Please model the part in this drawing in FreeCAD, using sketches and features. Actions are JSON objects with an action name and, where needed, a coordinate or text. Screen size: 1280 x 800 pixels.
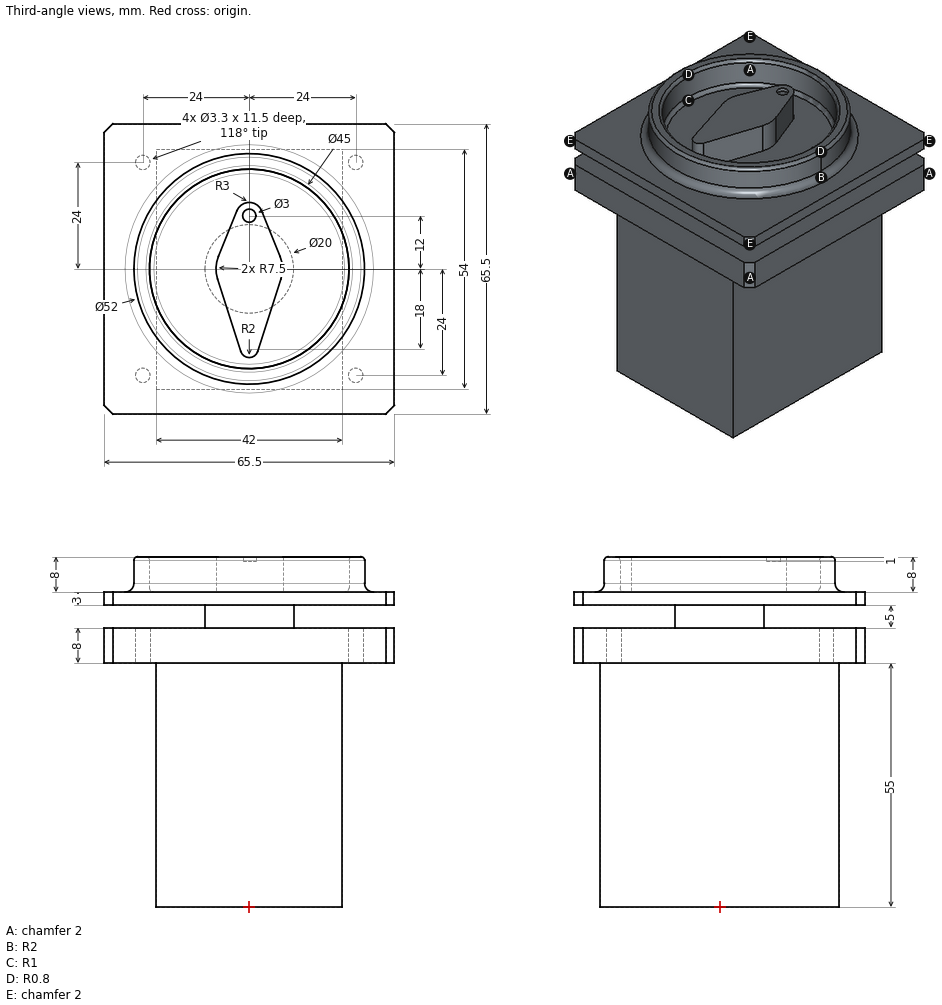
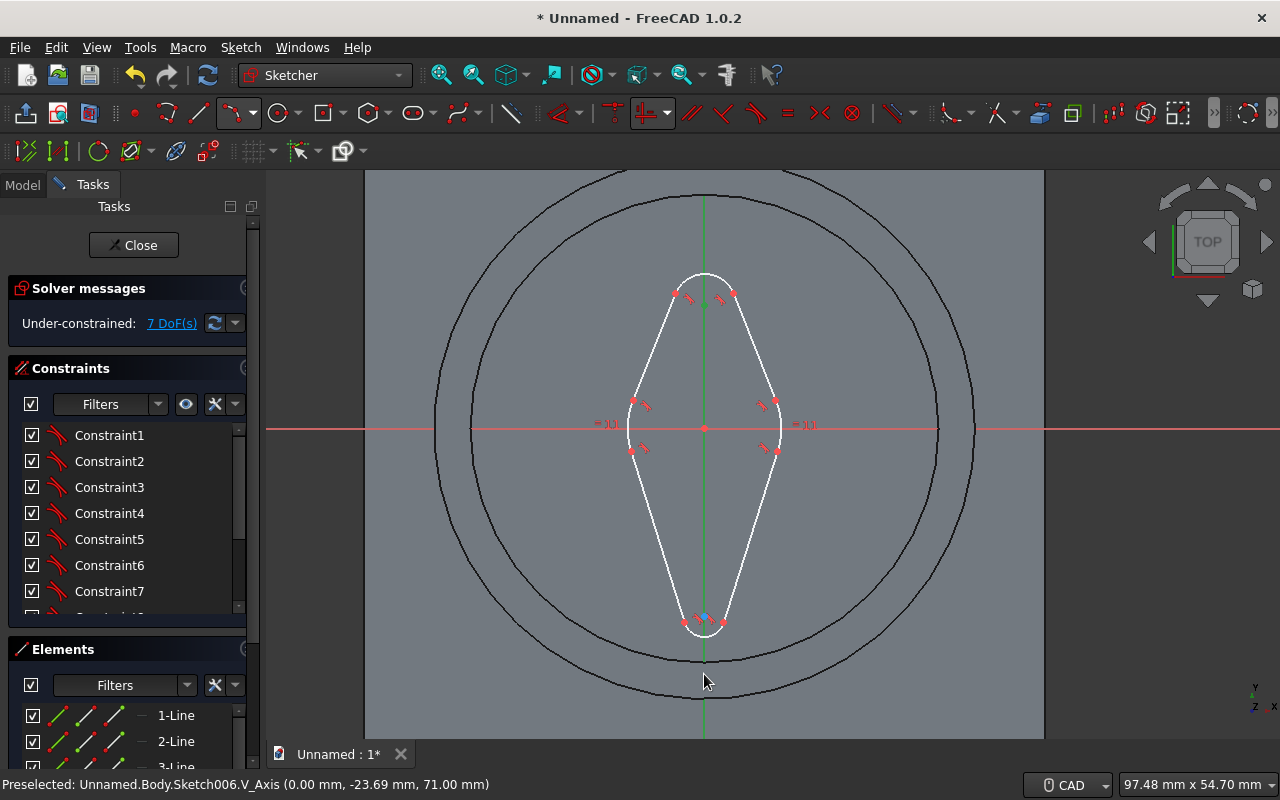
{"action": "left_click", "coordinate": [614, 114]}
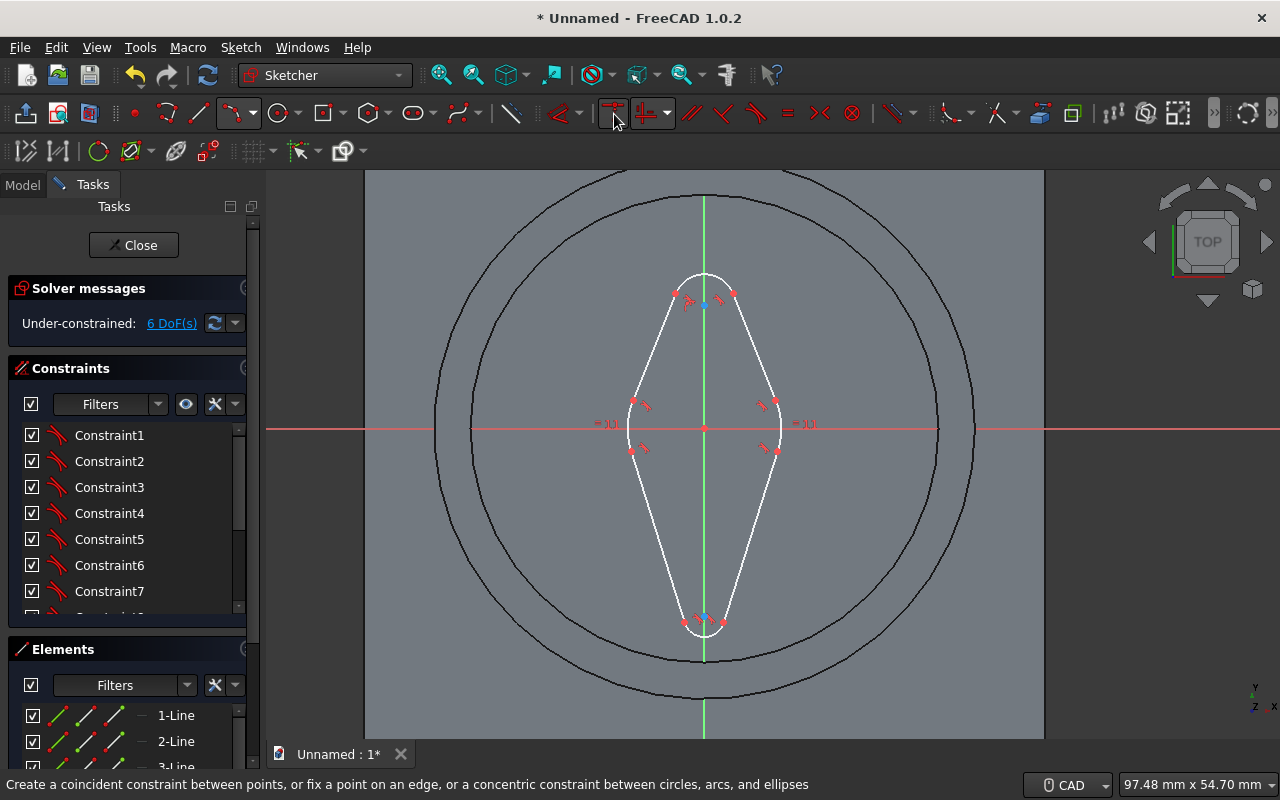
{"action": "left_click", "coordinate": [704, 617]}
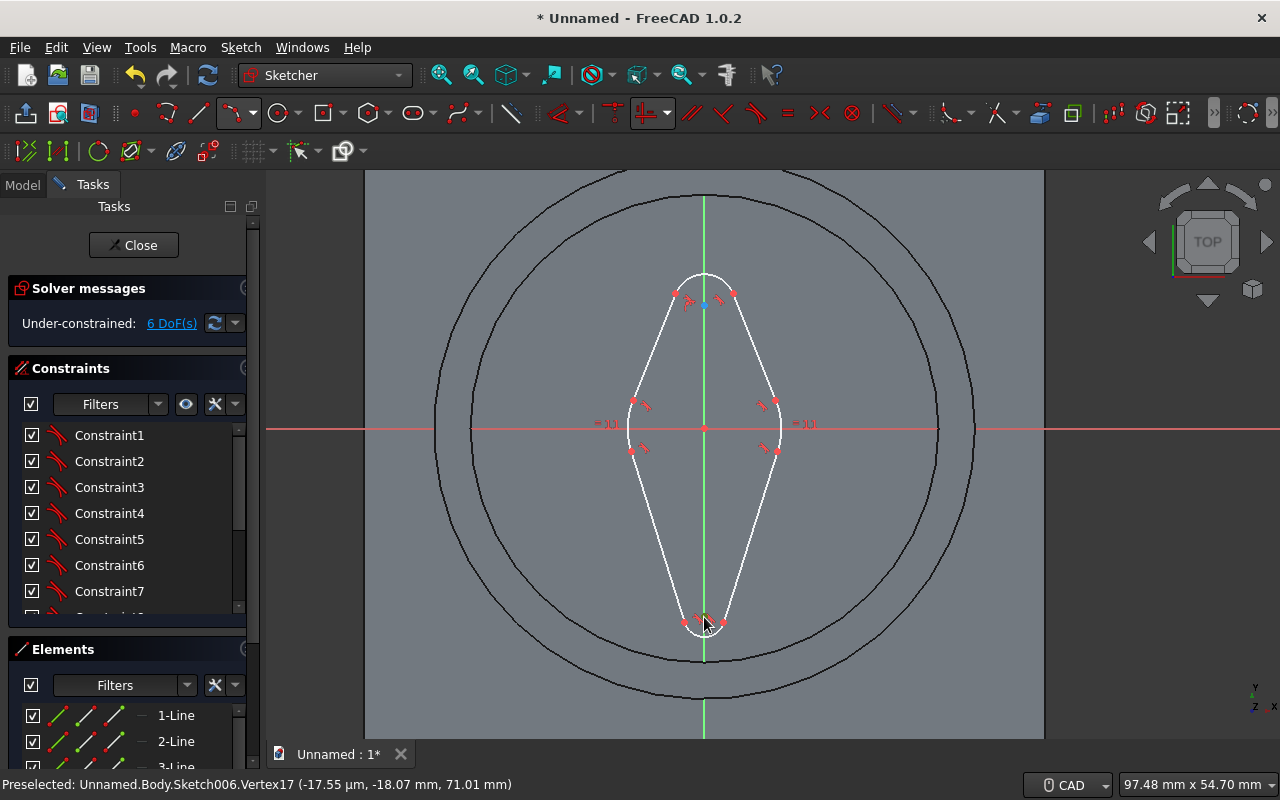
{"action": "left_click", "coordinate": [704, 674]}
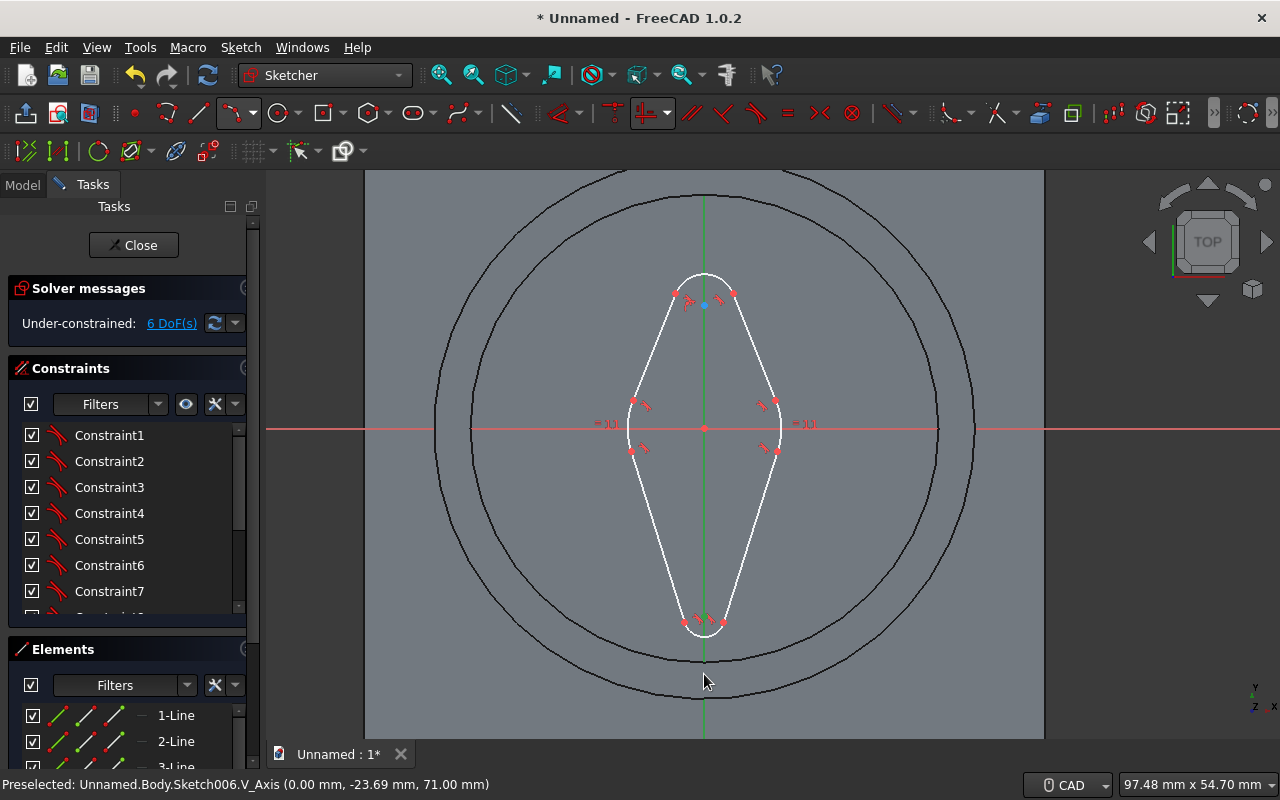
{"action": "left_click", "coordinate": [614, 114]}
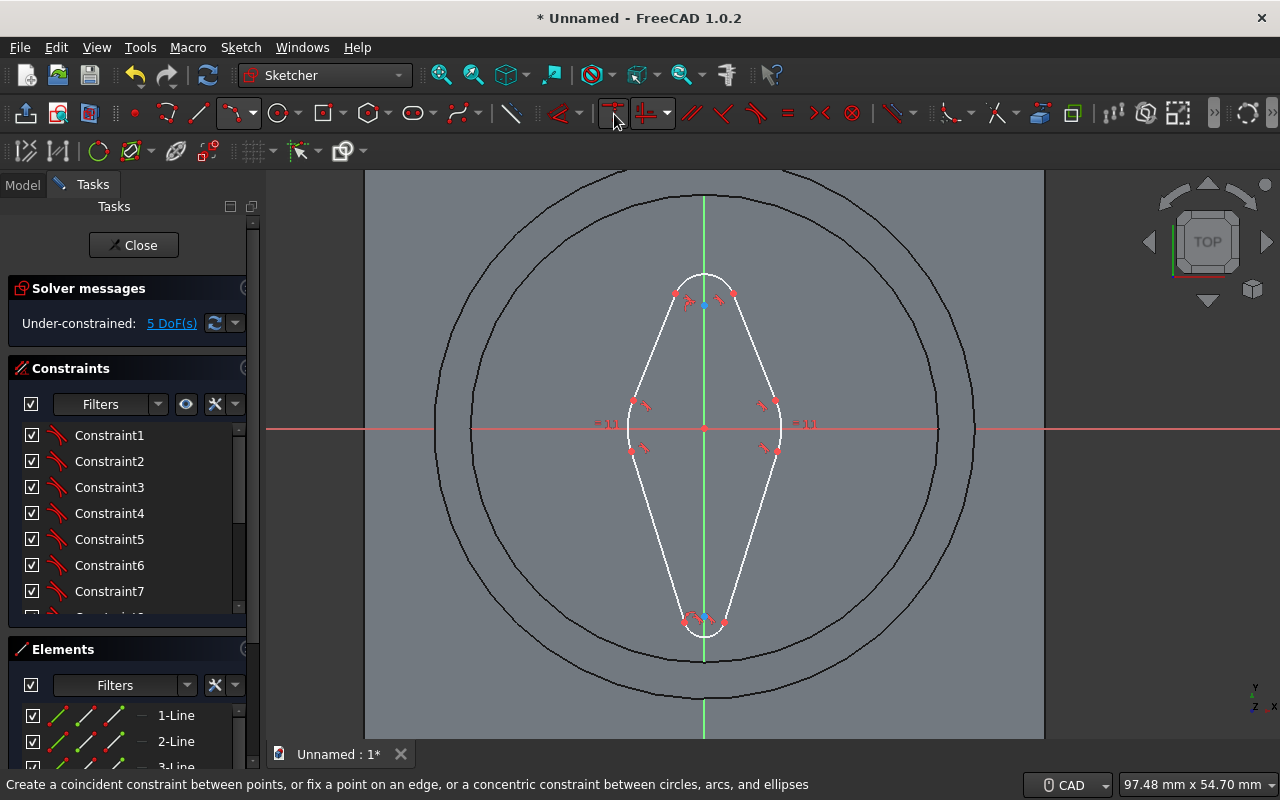
{"action": "left_click", "coordinate": [558, 114]}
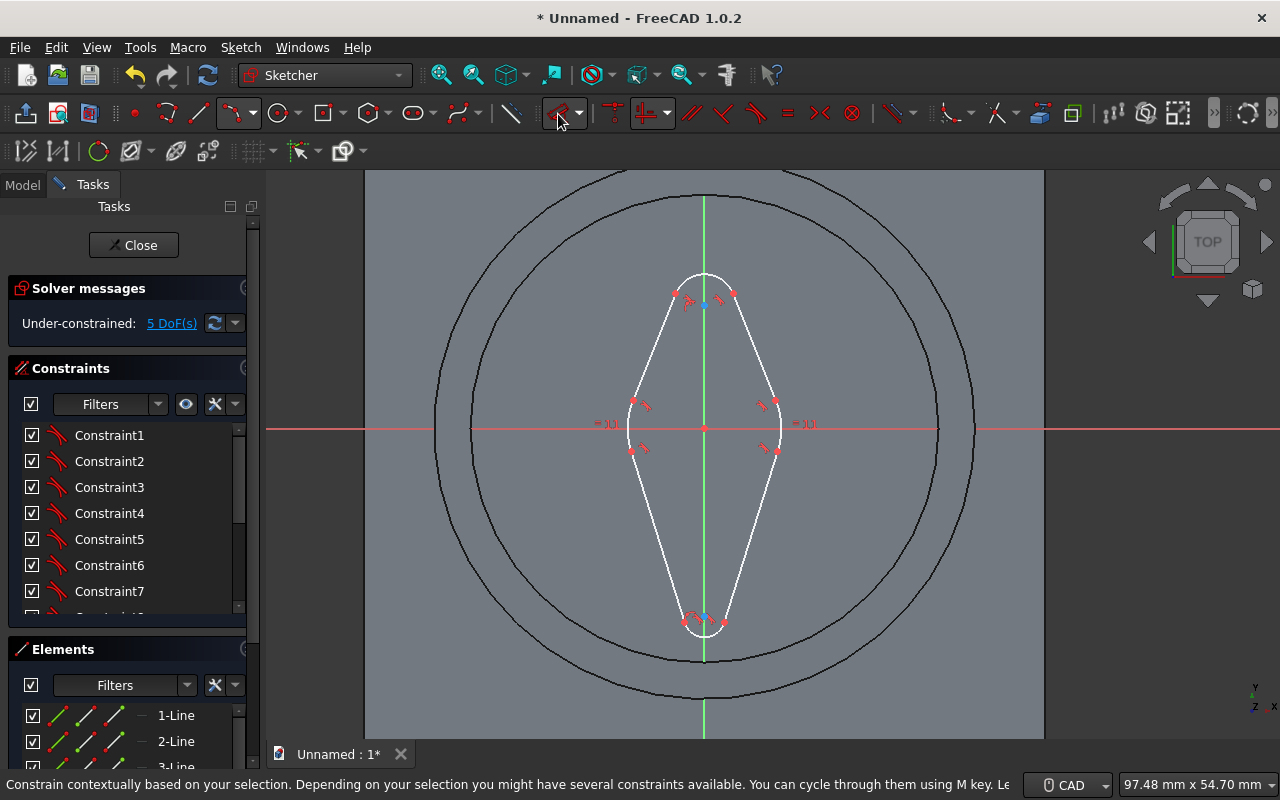
{"action": "scroll", "coordinate": [719, 278], "scroll_direction": "up", "scroll_amount": 2}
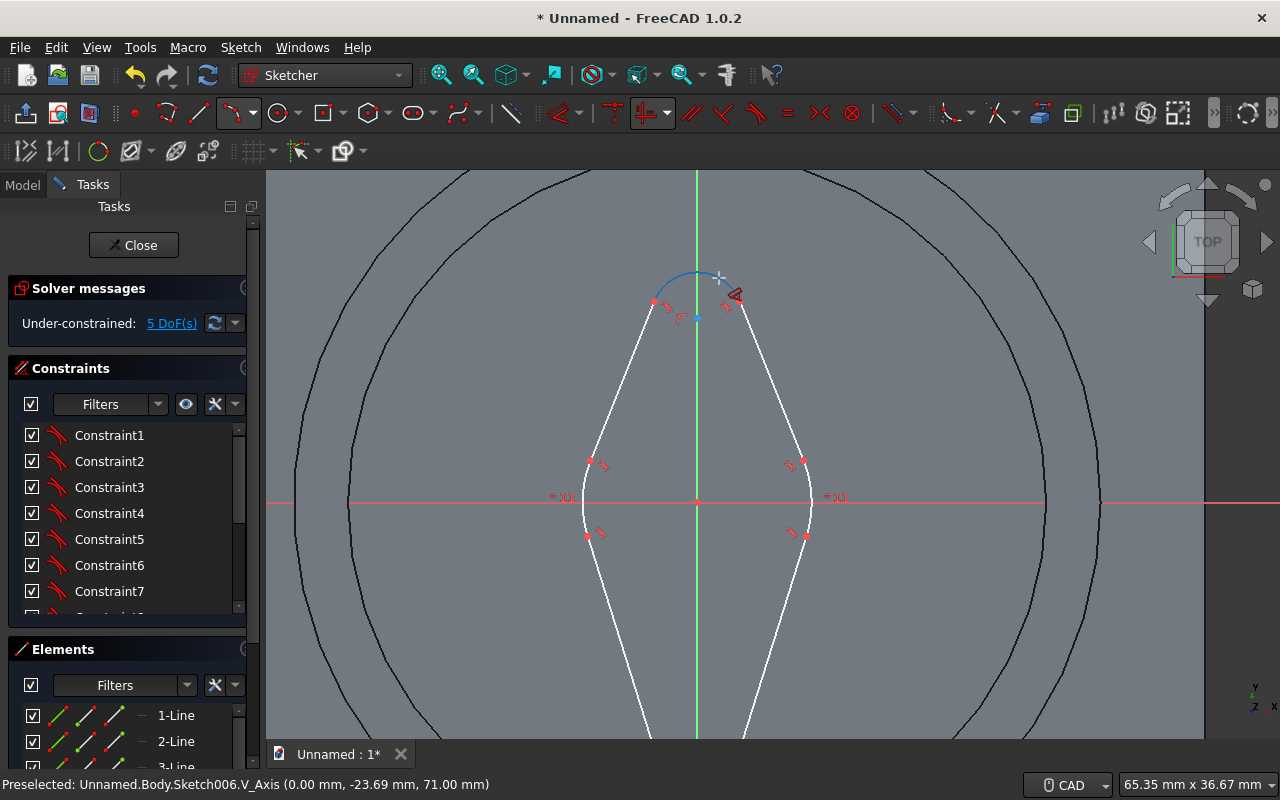
{"action": "left_click", "coordinate": [718, 278]}
{"action": "left_click", "coordinate": [733, 250]}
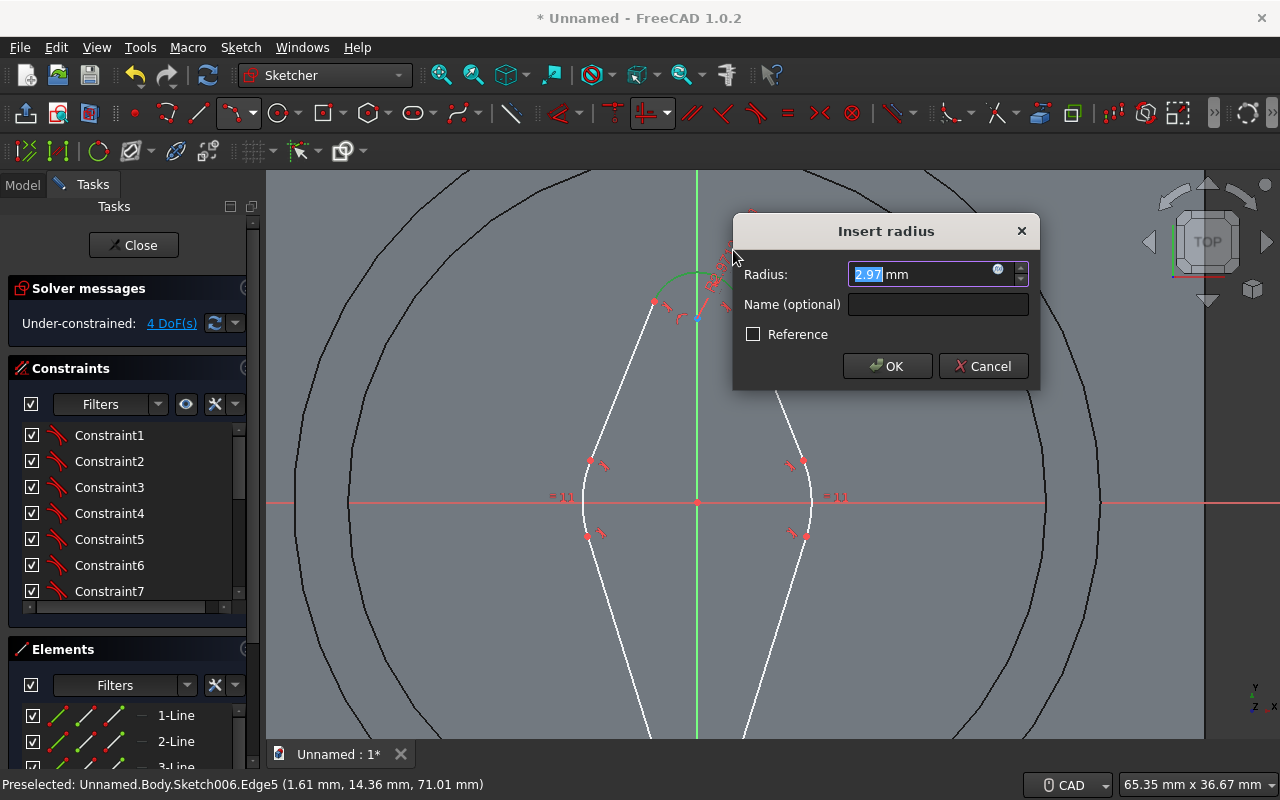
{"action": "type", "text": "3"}
{"action": "key", "text": "Return"}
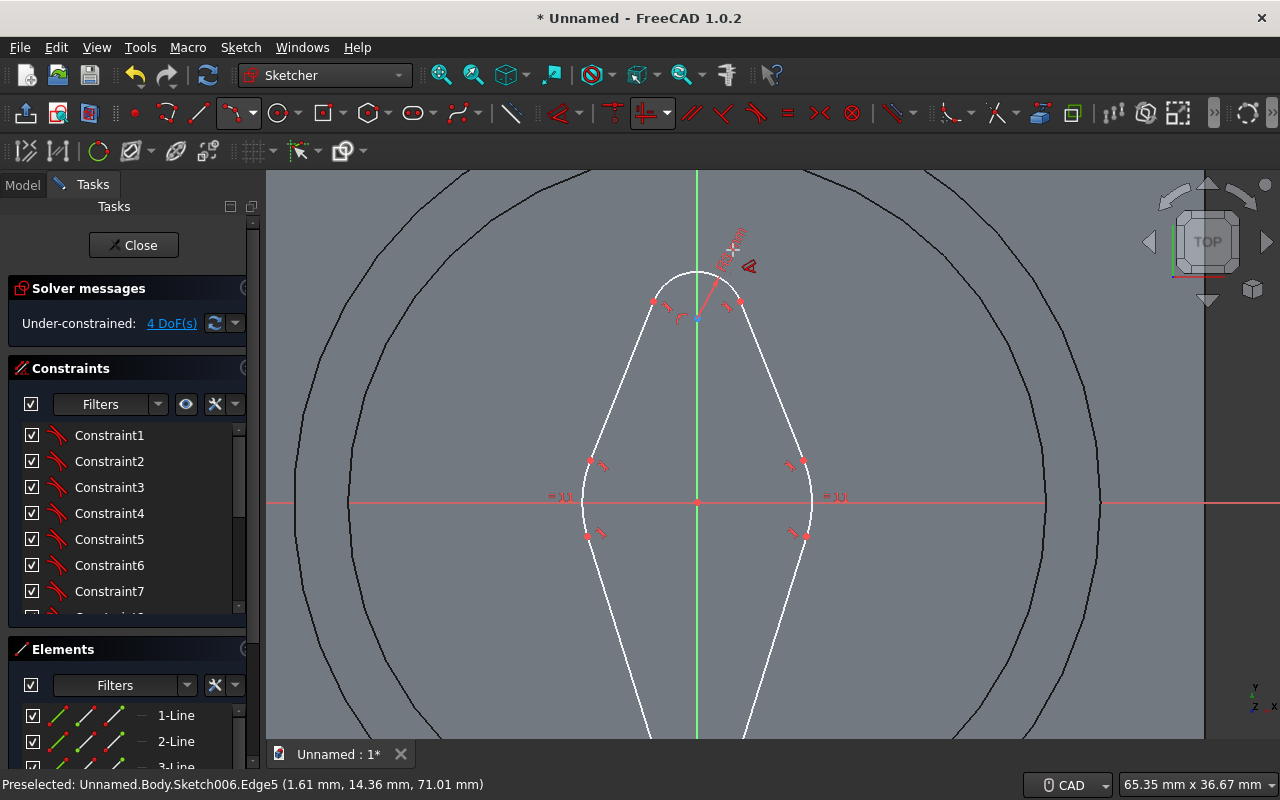
{"action": "left_click", "coordinate": [584, 483]}
{"action": "left_click", "coordinate": [552, 478]}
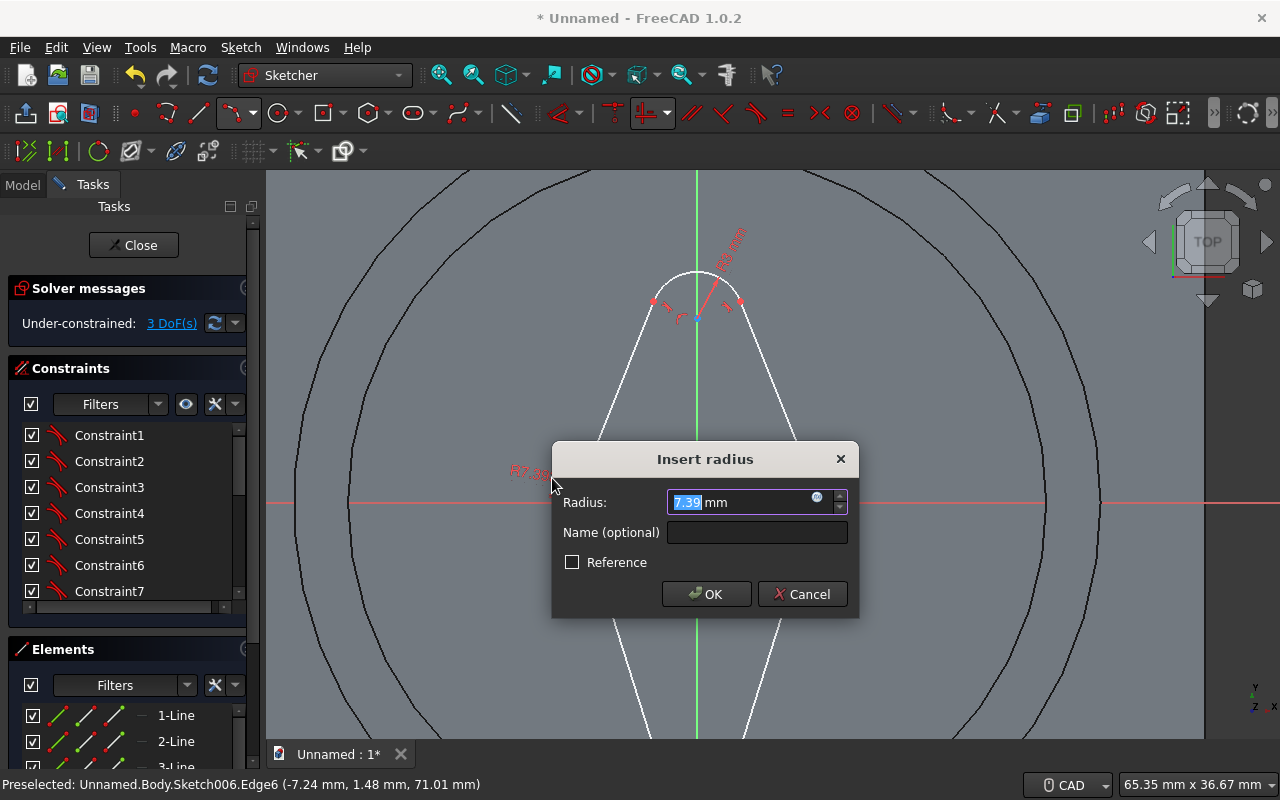
{"action": "type", "text": "7.5"}
{"action": "key", "text": "Return"}